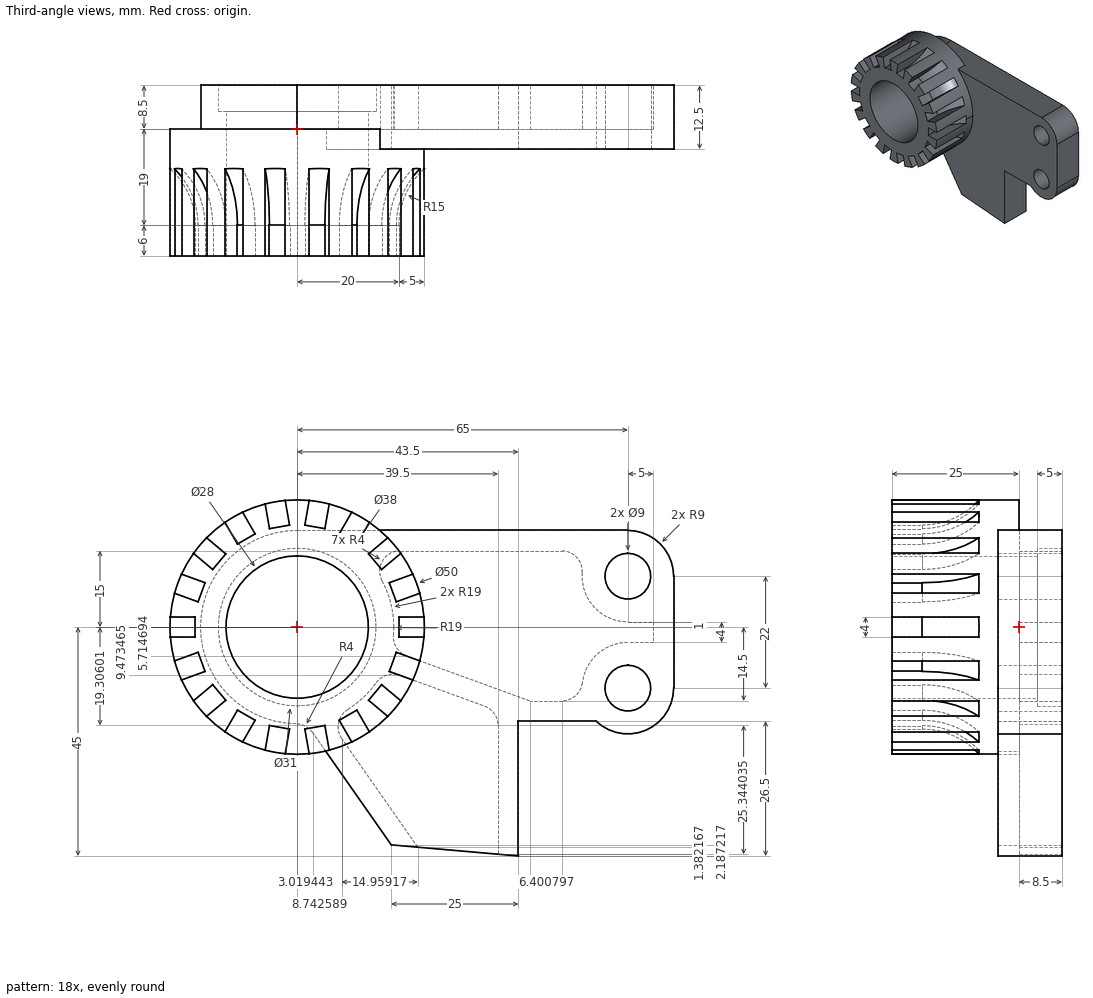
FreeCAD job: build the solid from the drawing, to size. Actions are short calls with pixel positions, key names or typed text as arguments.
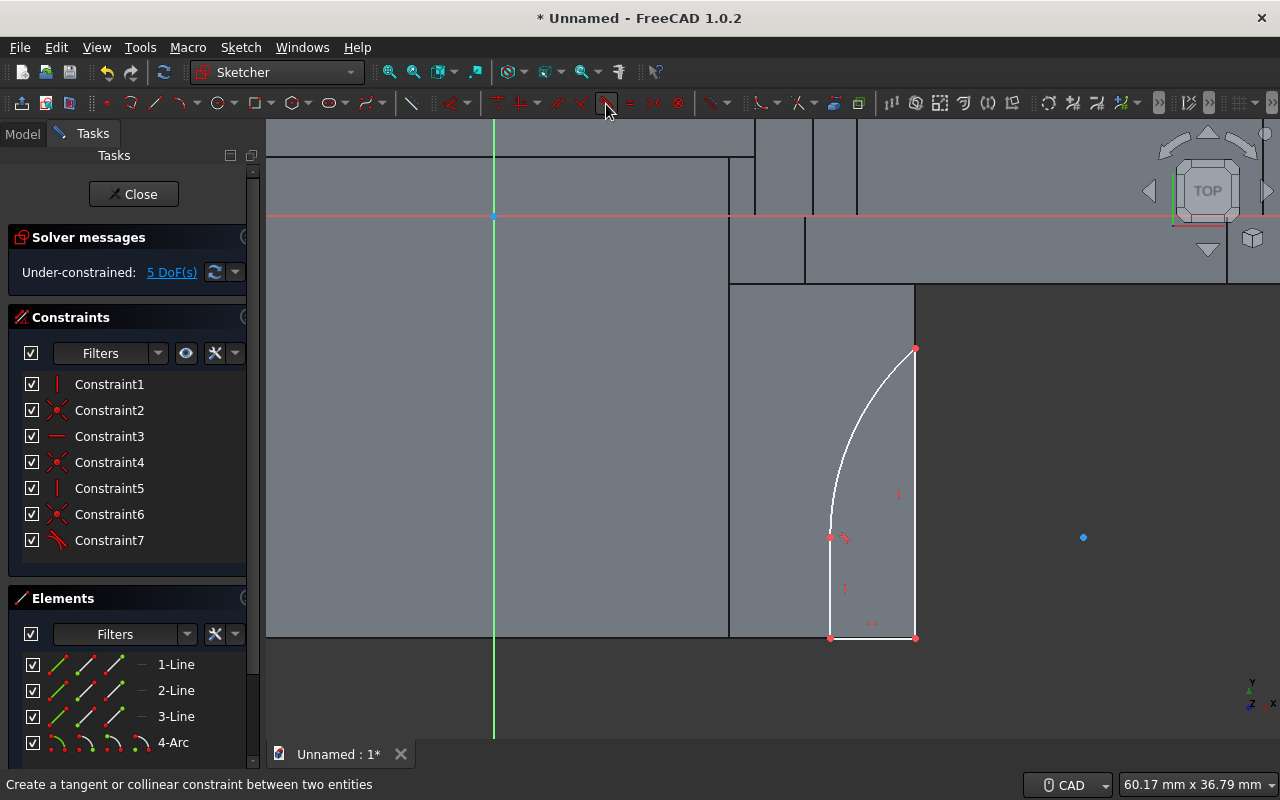
click(450, 104)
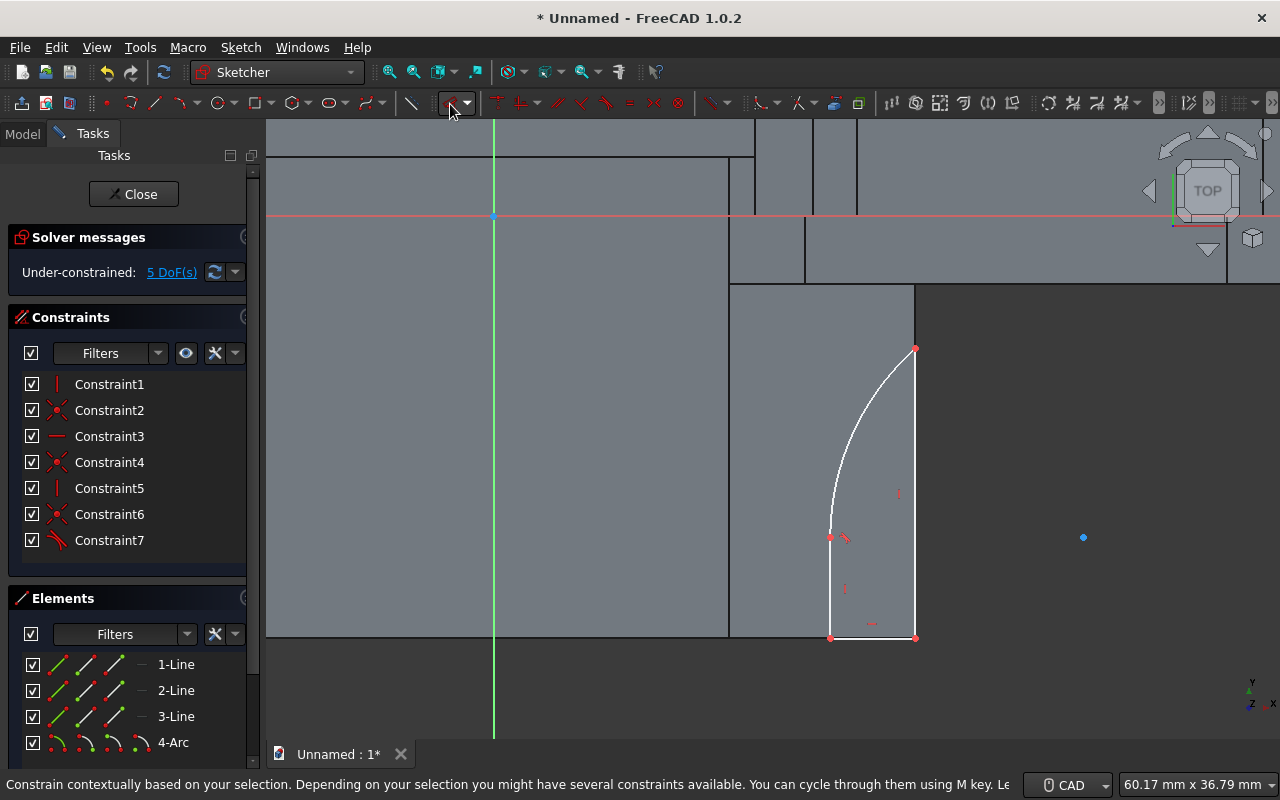
click(873, 397)
click(846, 379)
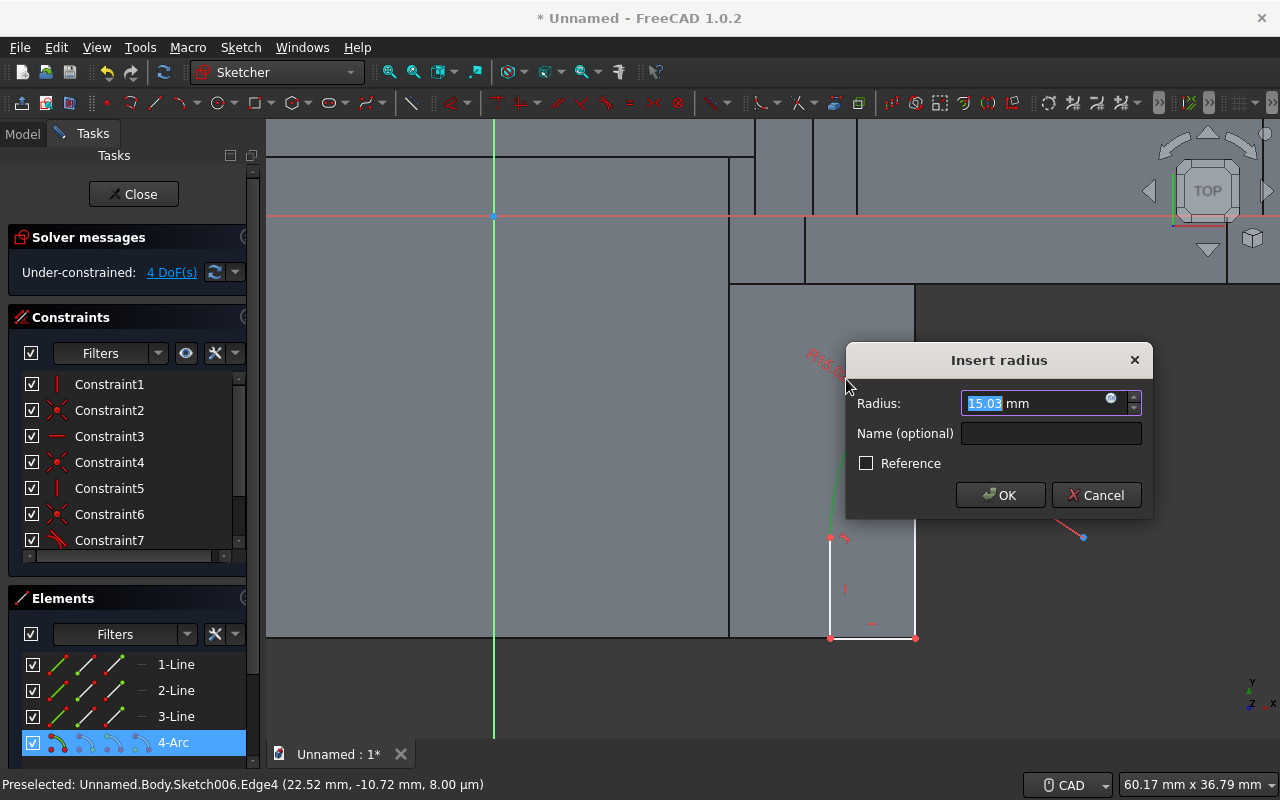
text(15)
key(Return)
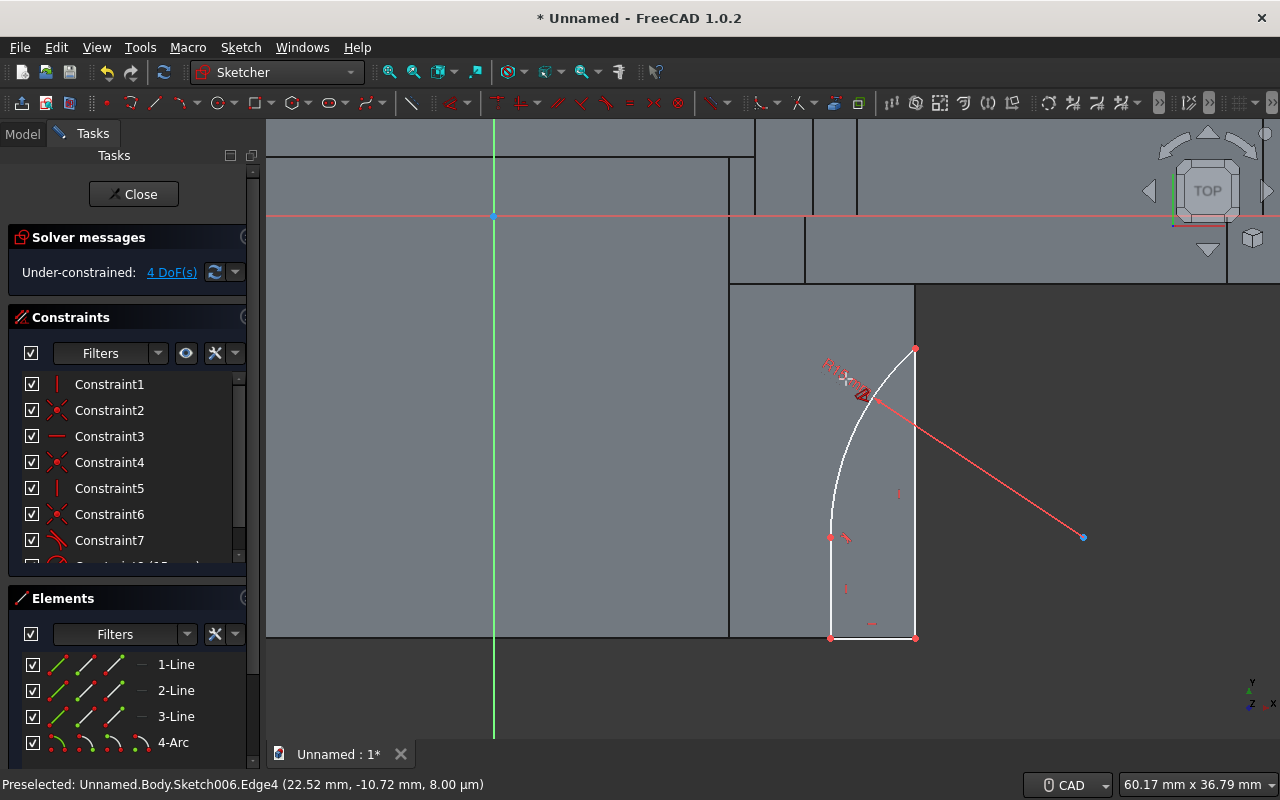
click(831, 568)
click(865, 588)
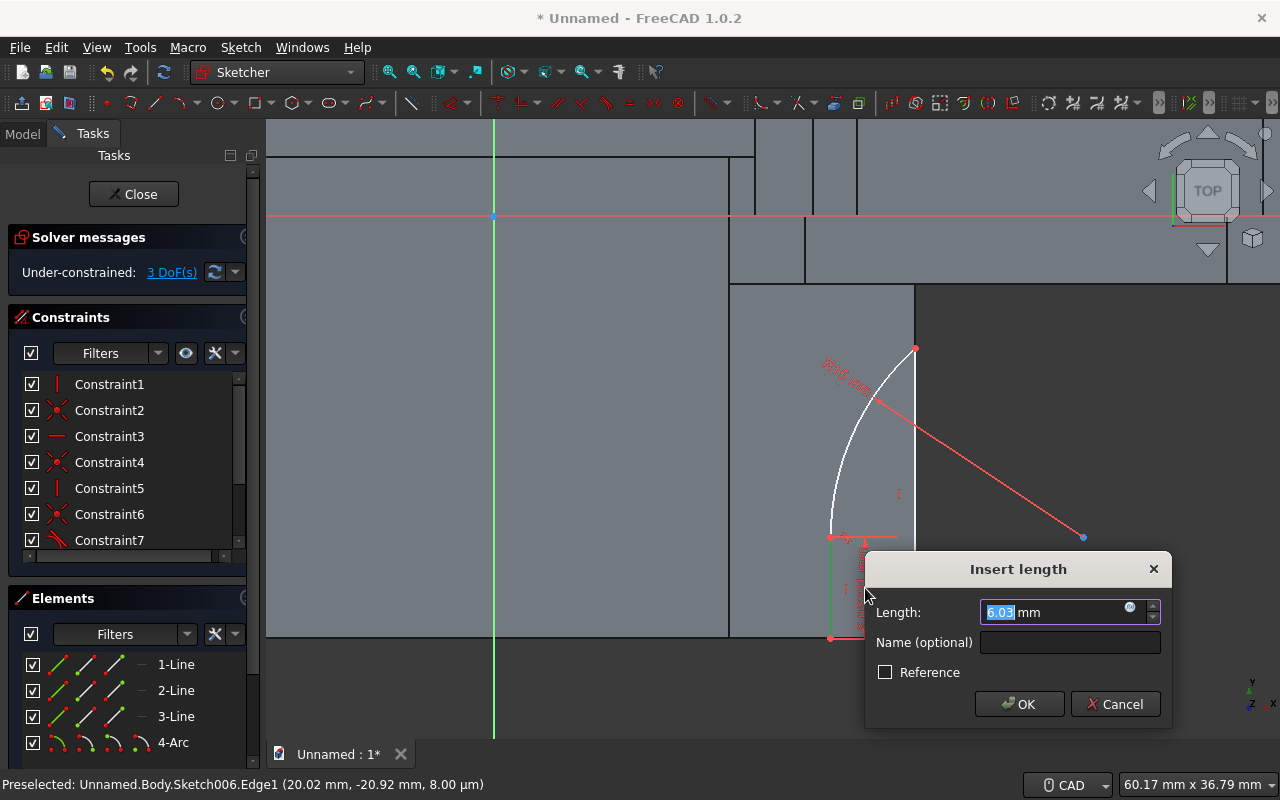
text(6)
key(Return)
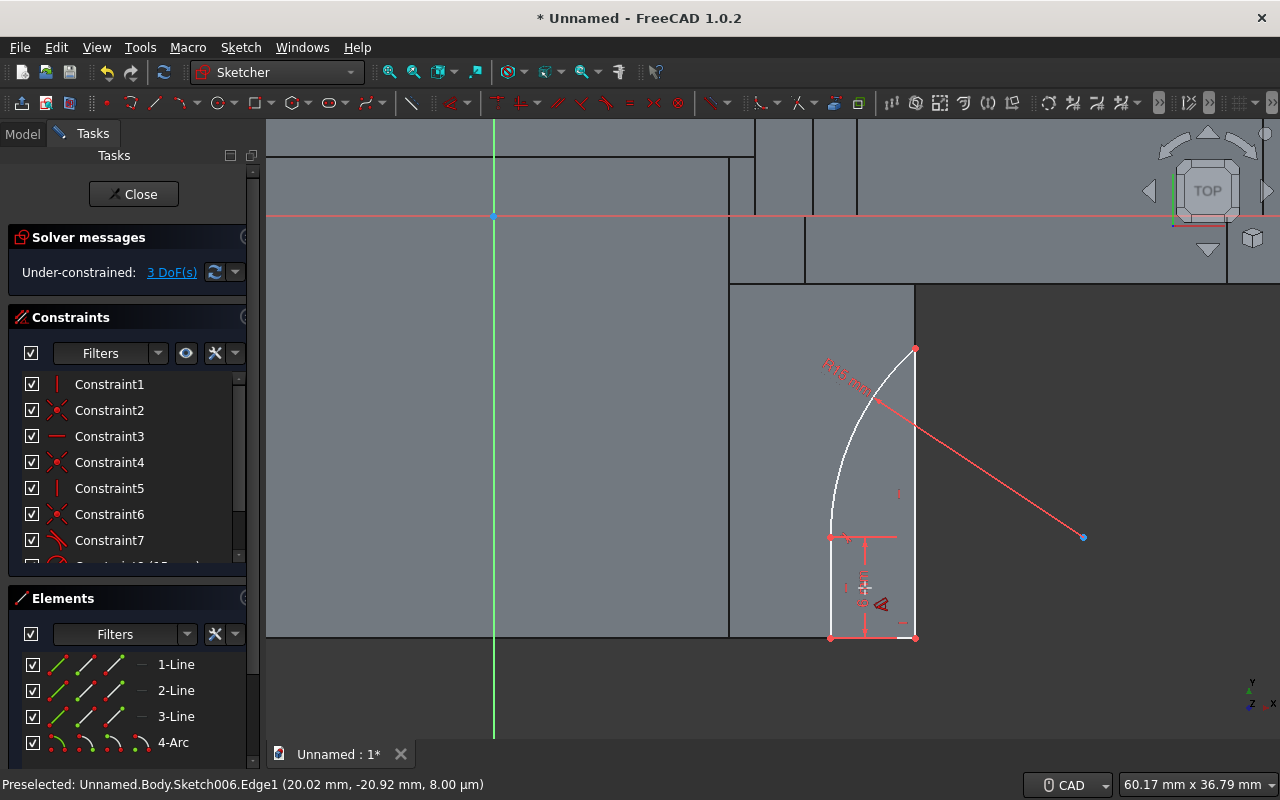
click(856, 638)
click(873, 672)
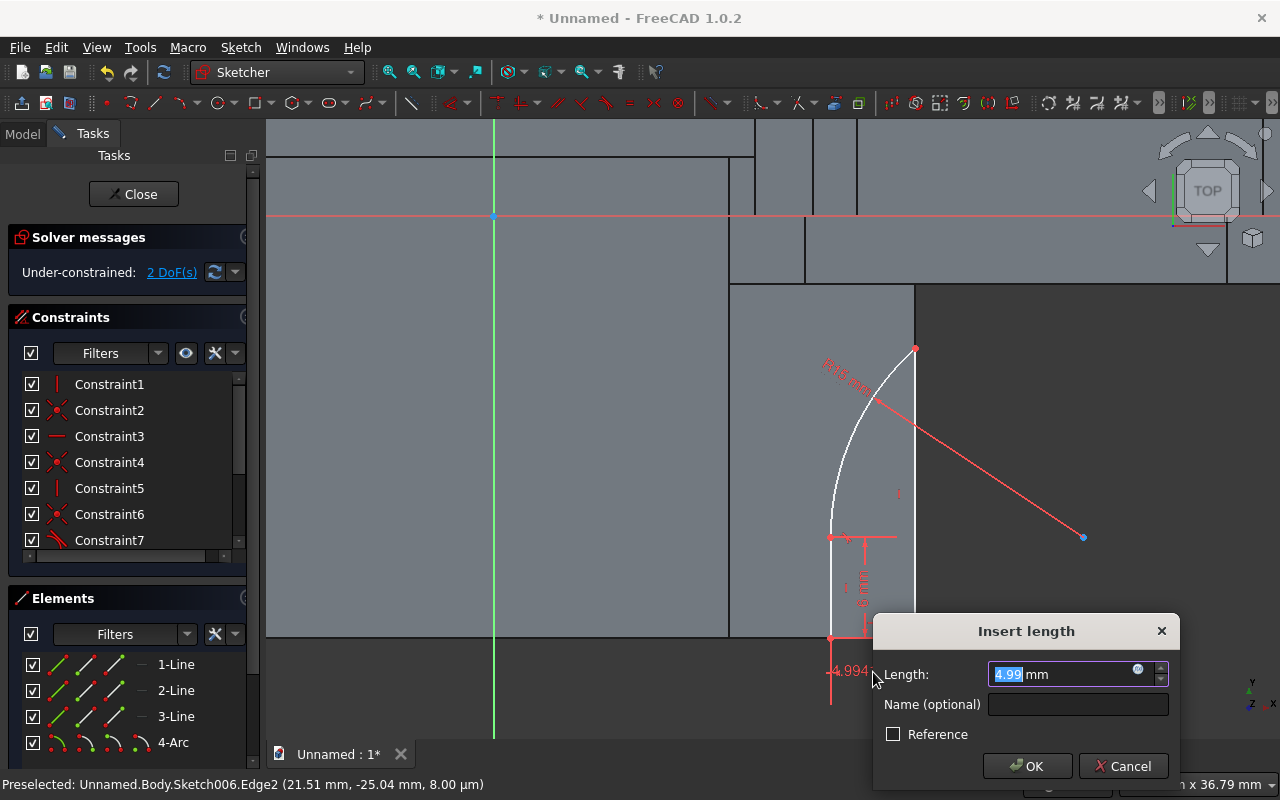
text(5)
key(Return)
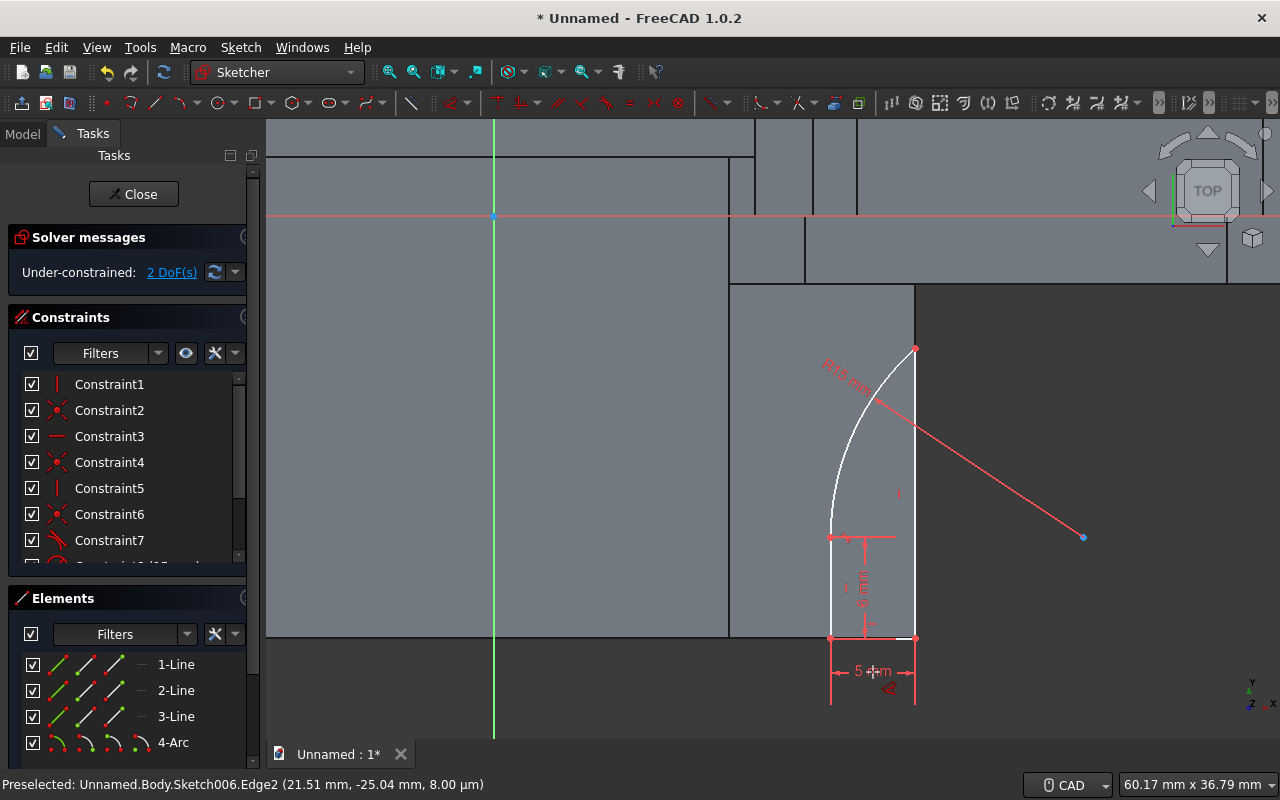
click(831, 537)
click(662, 182)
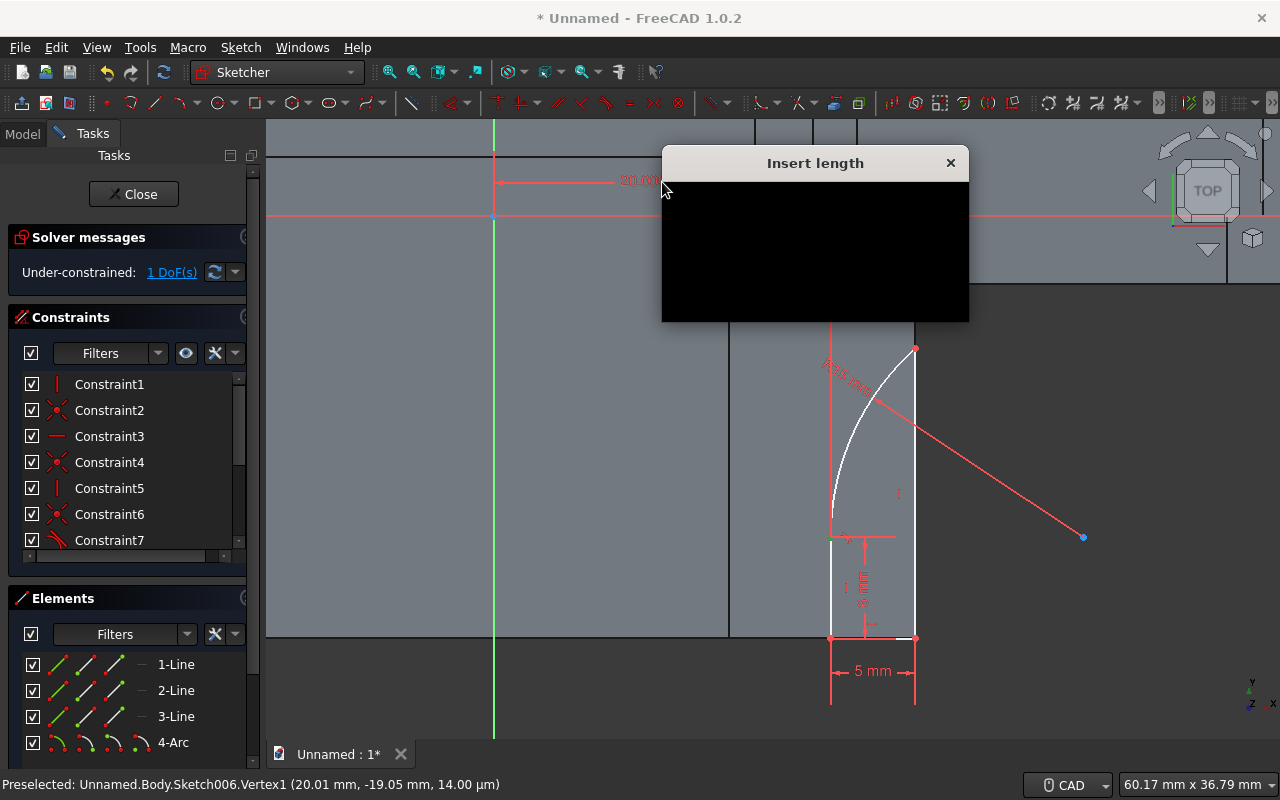
text(20)
key(Return)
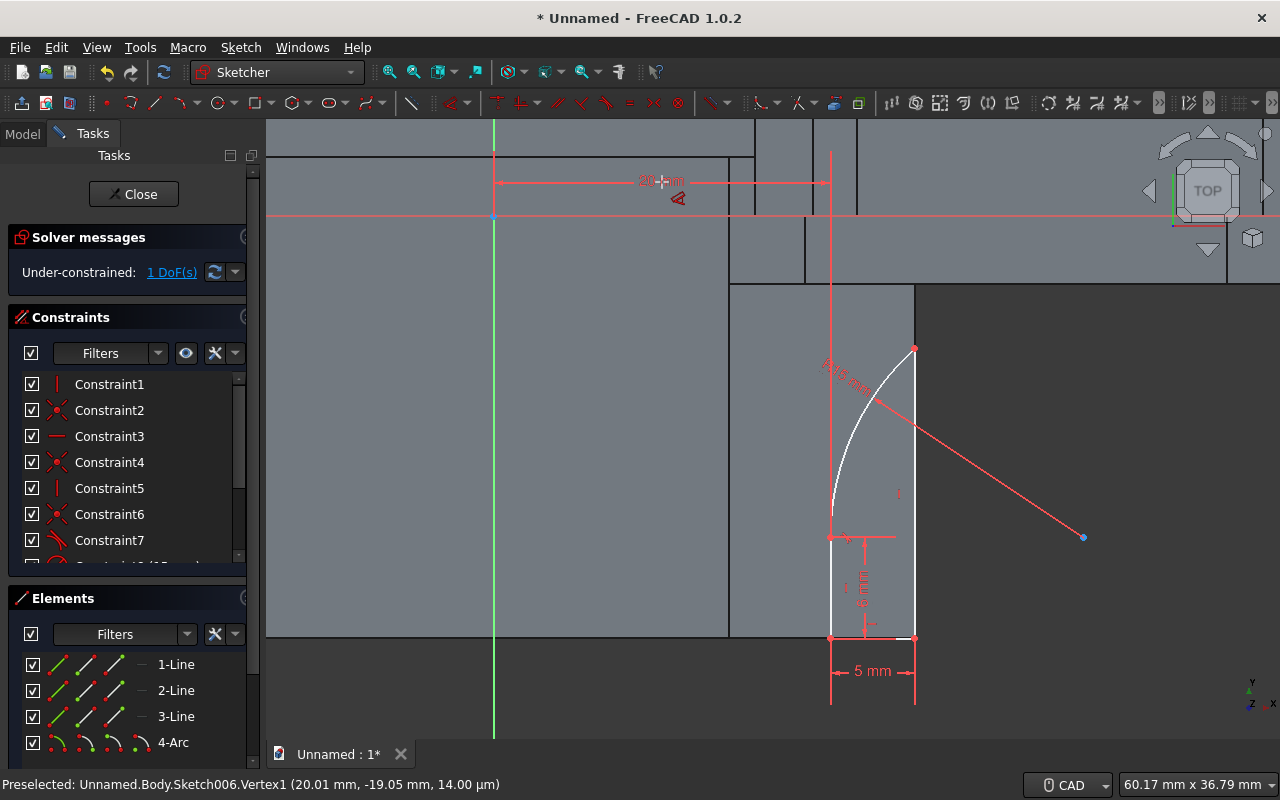
click(831, 537)
click(460, 377)